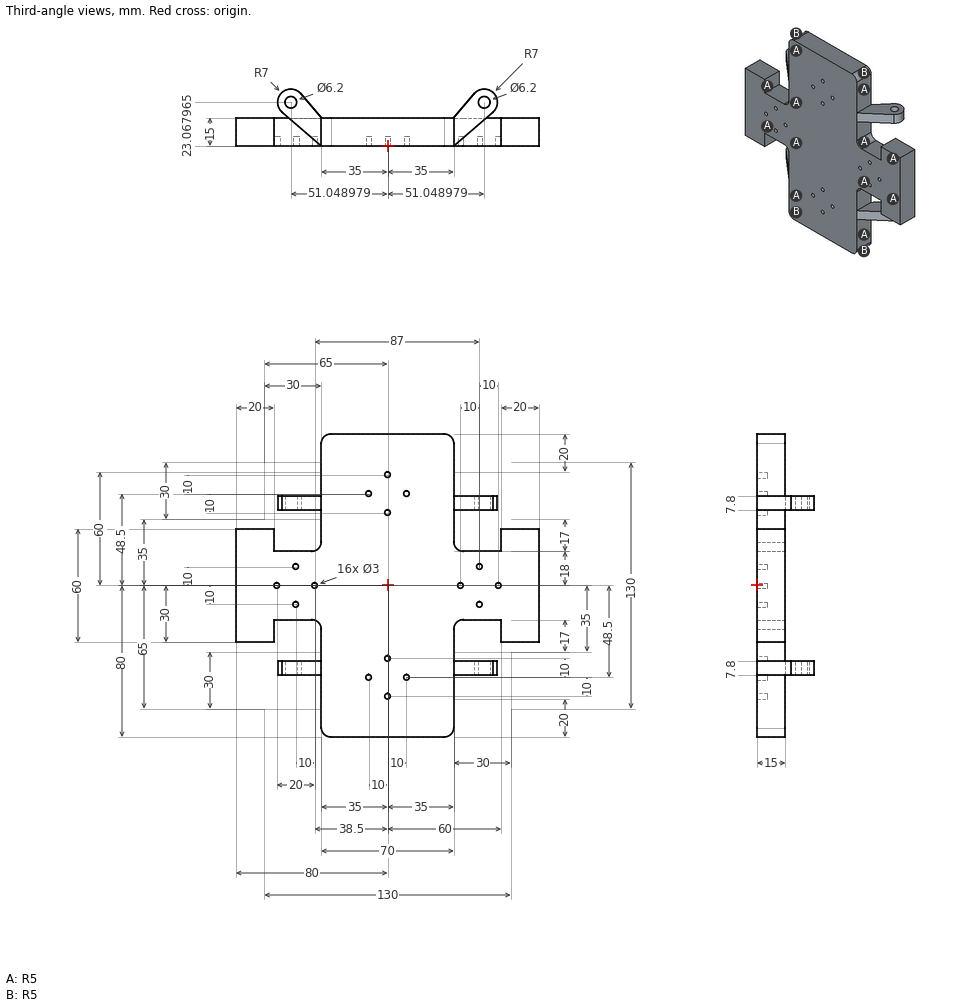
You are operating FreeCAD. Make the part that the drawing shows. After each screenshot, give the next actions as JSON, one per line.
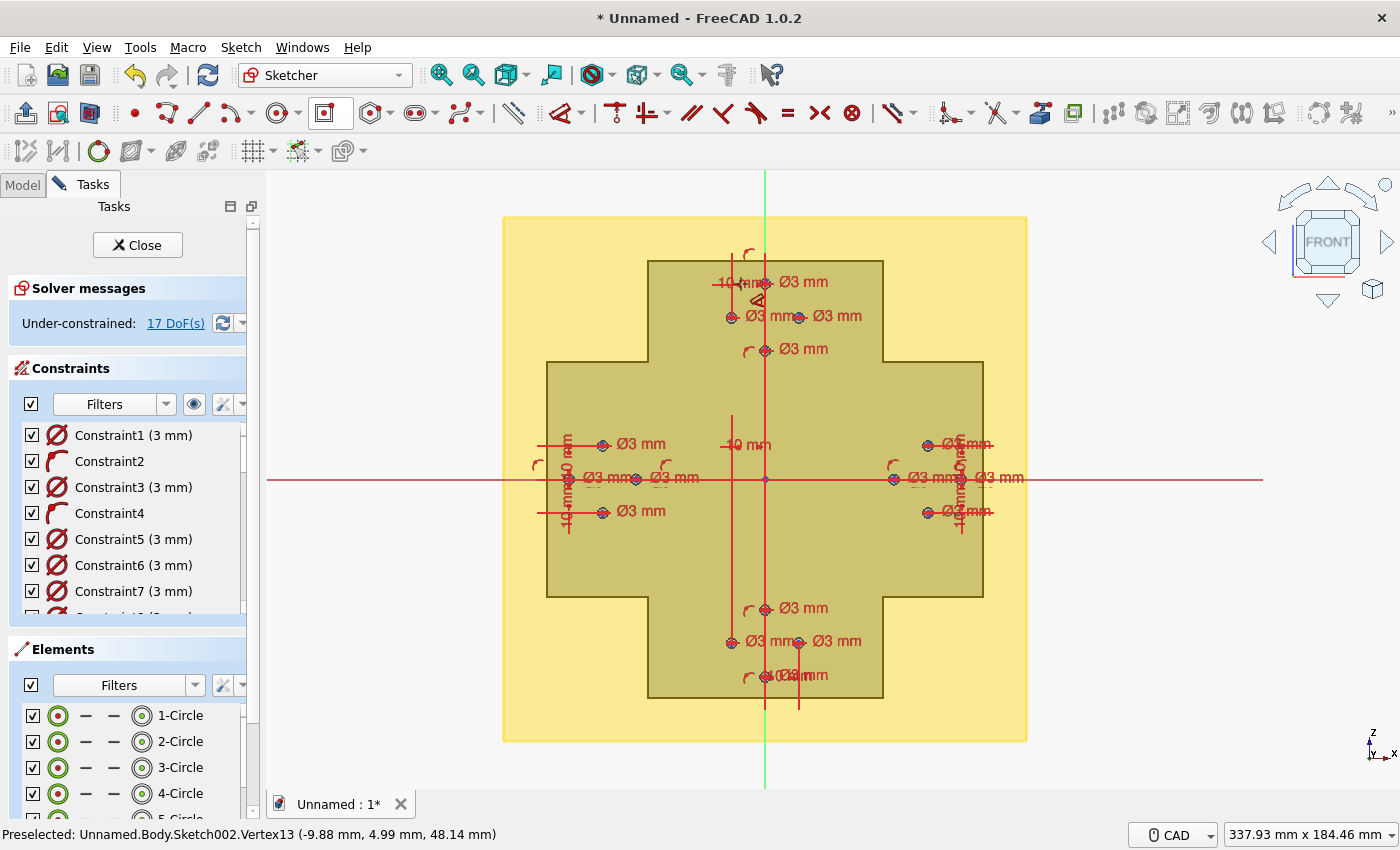
{"action": "left_click", "coordinate": [799, 318]}
{"action": "left_click", "coordinate": [782, 514]}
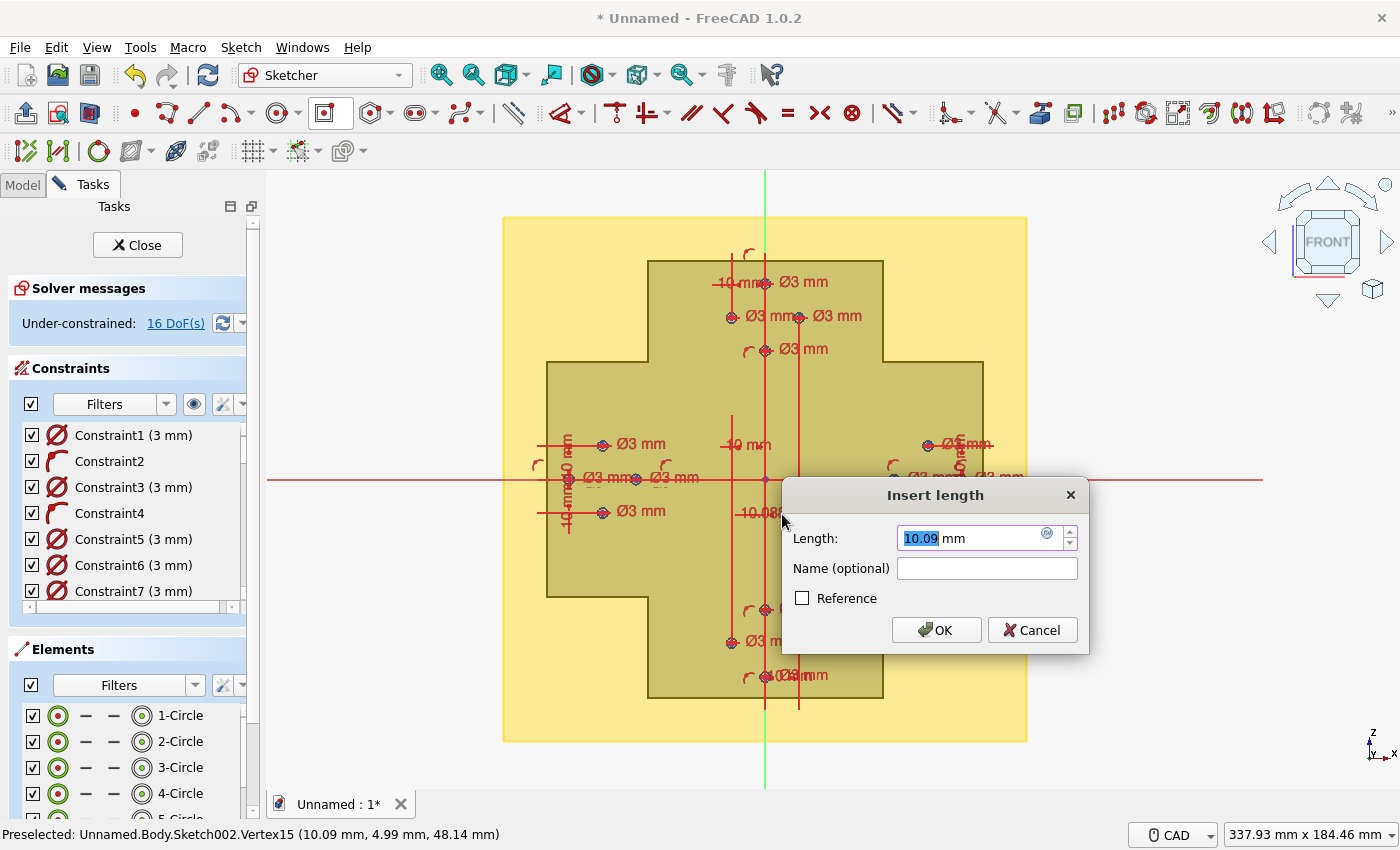
{"action": "type", "text": "10"}
{"action": "key", "text": "Return"}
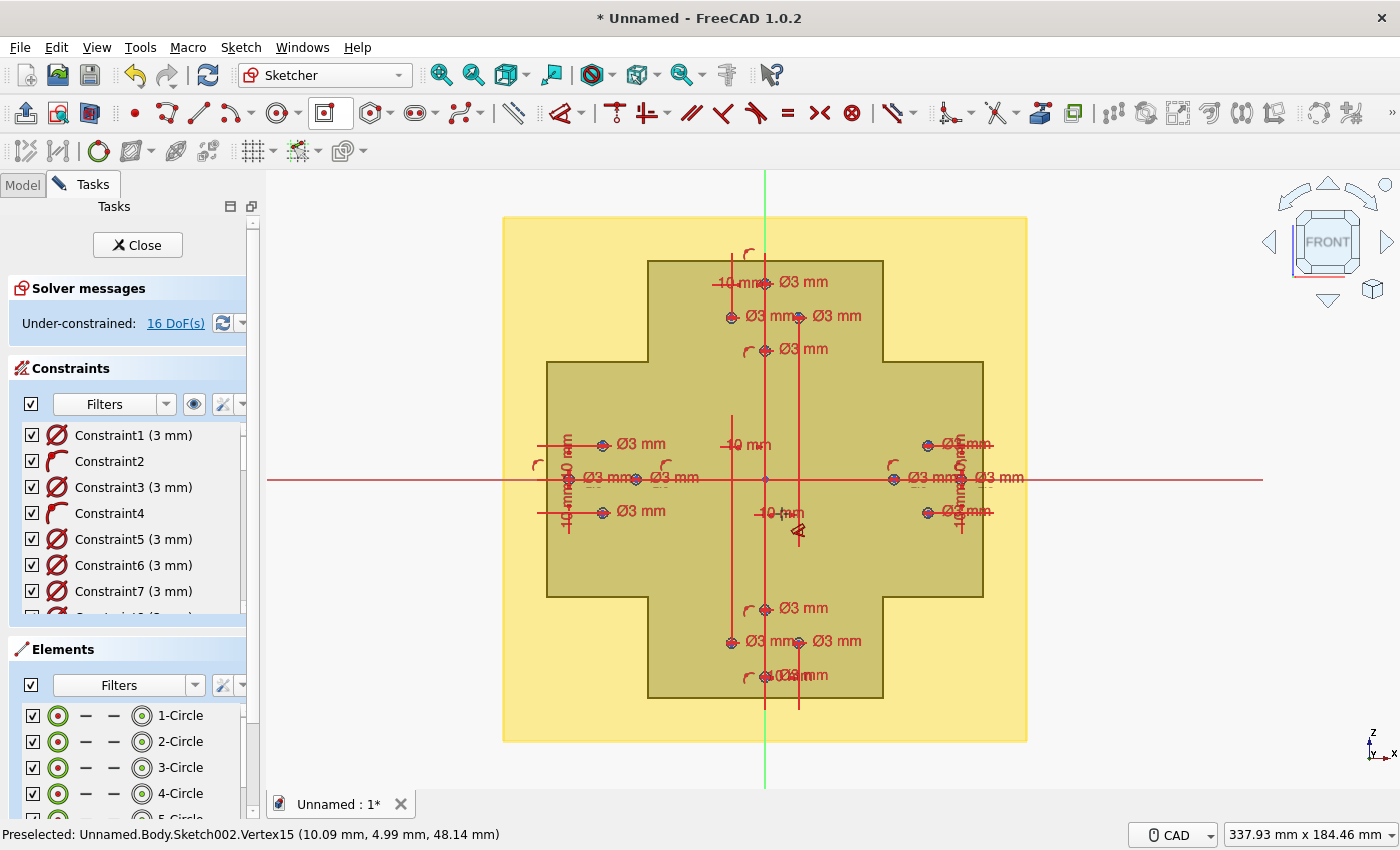
{"action": "left_click", "coordinate": [636, 480]}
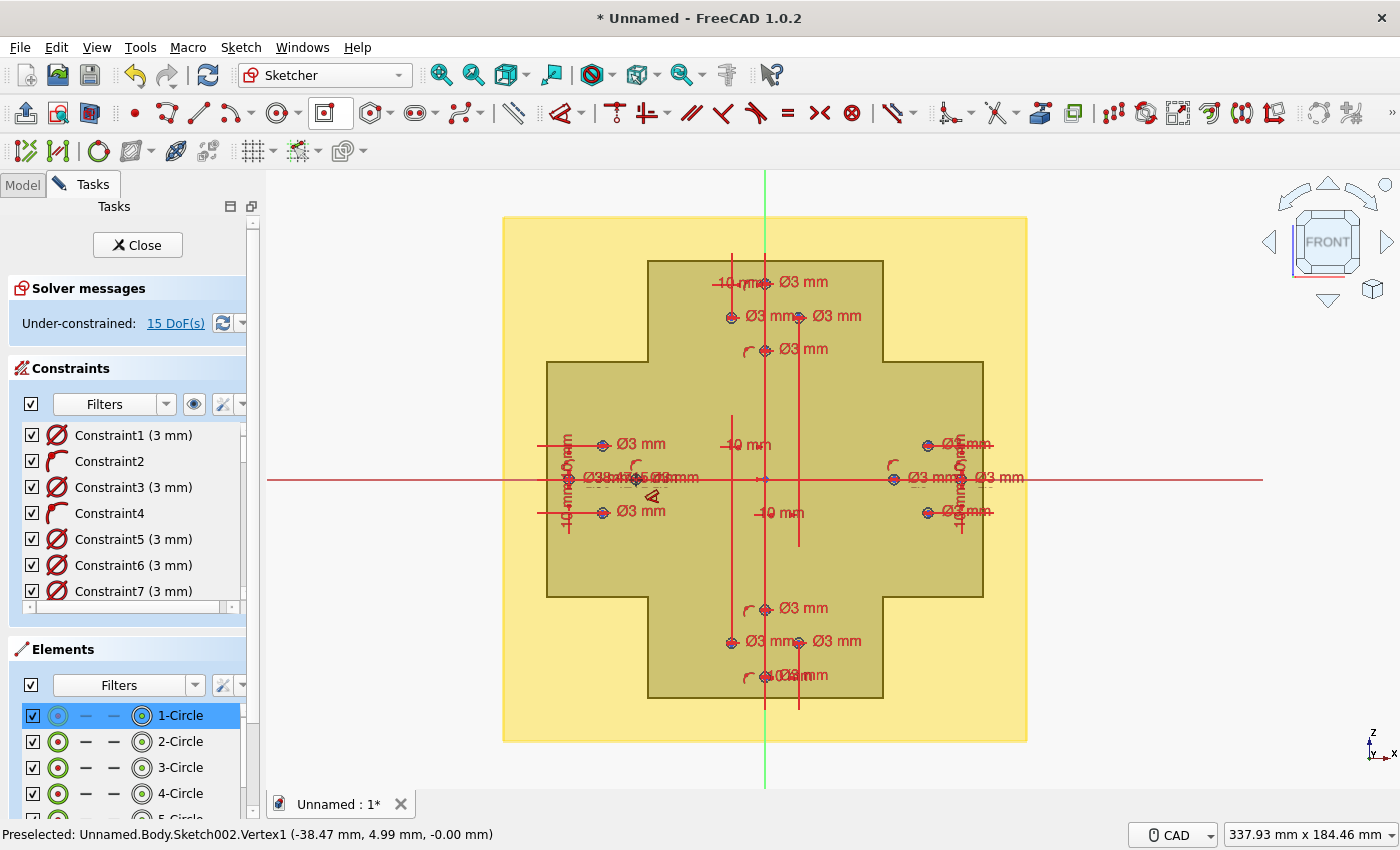
{"action": "left_click", "coordinate": [569, 480]}
{"action": "left_click", "coordinate": [603, 538]}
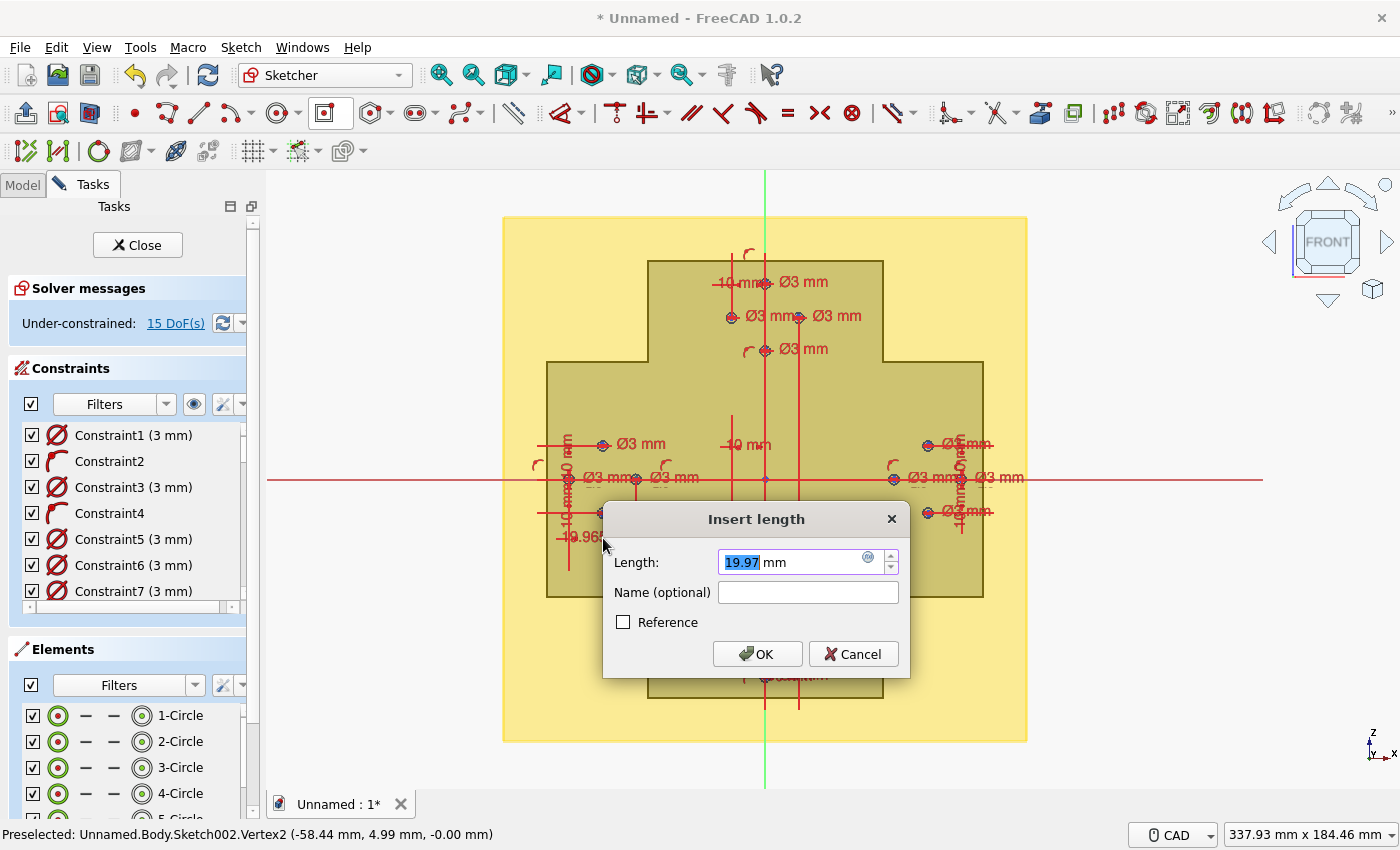
{"action": "type", "text": "20"}
{"action": "key", "text": "Return"}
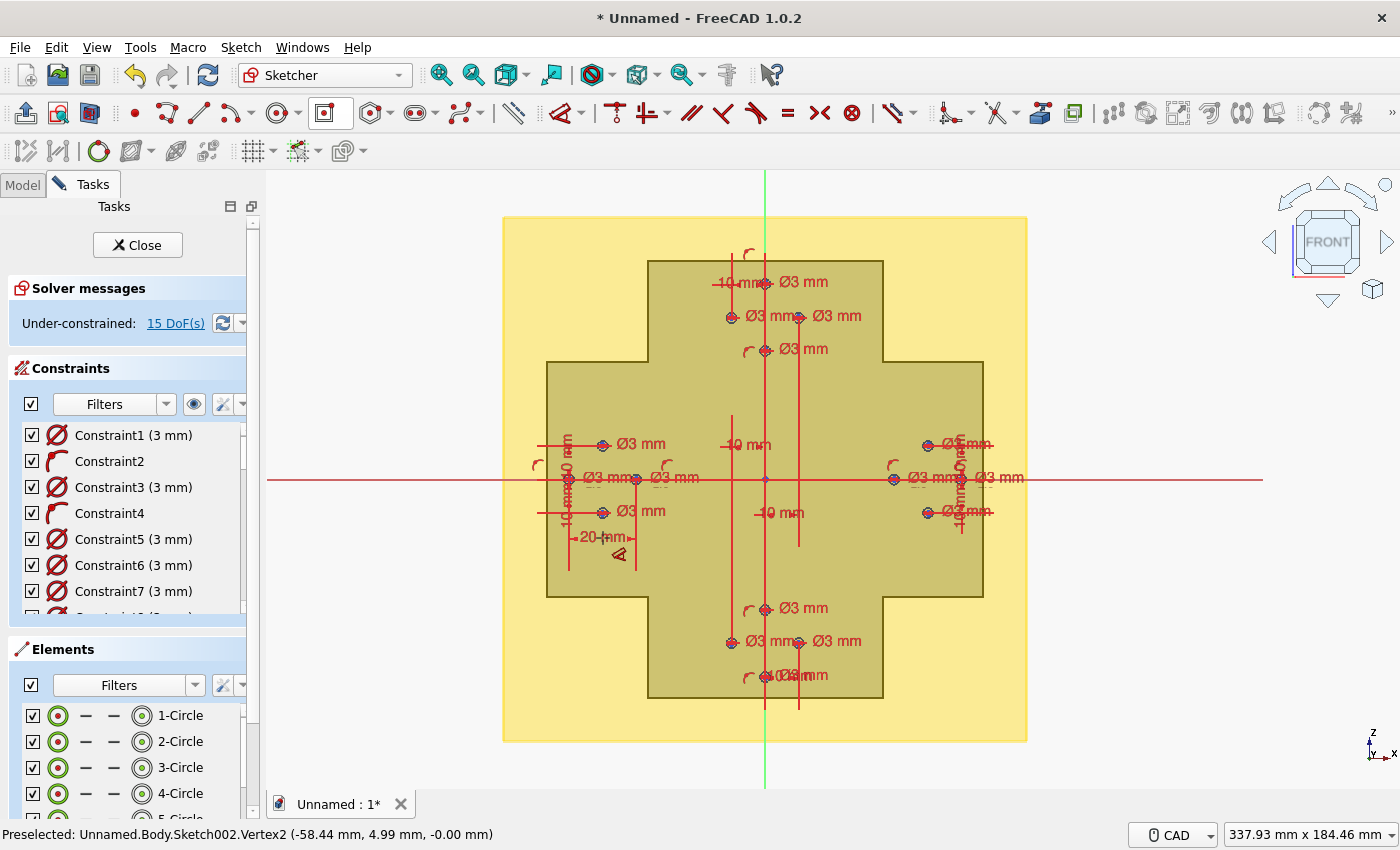
{"action": "left_click", "coordinate": [636, 480]}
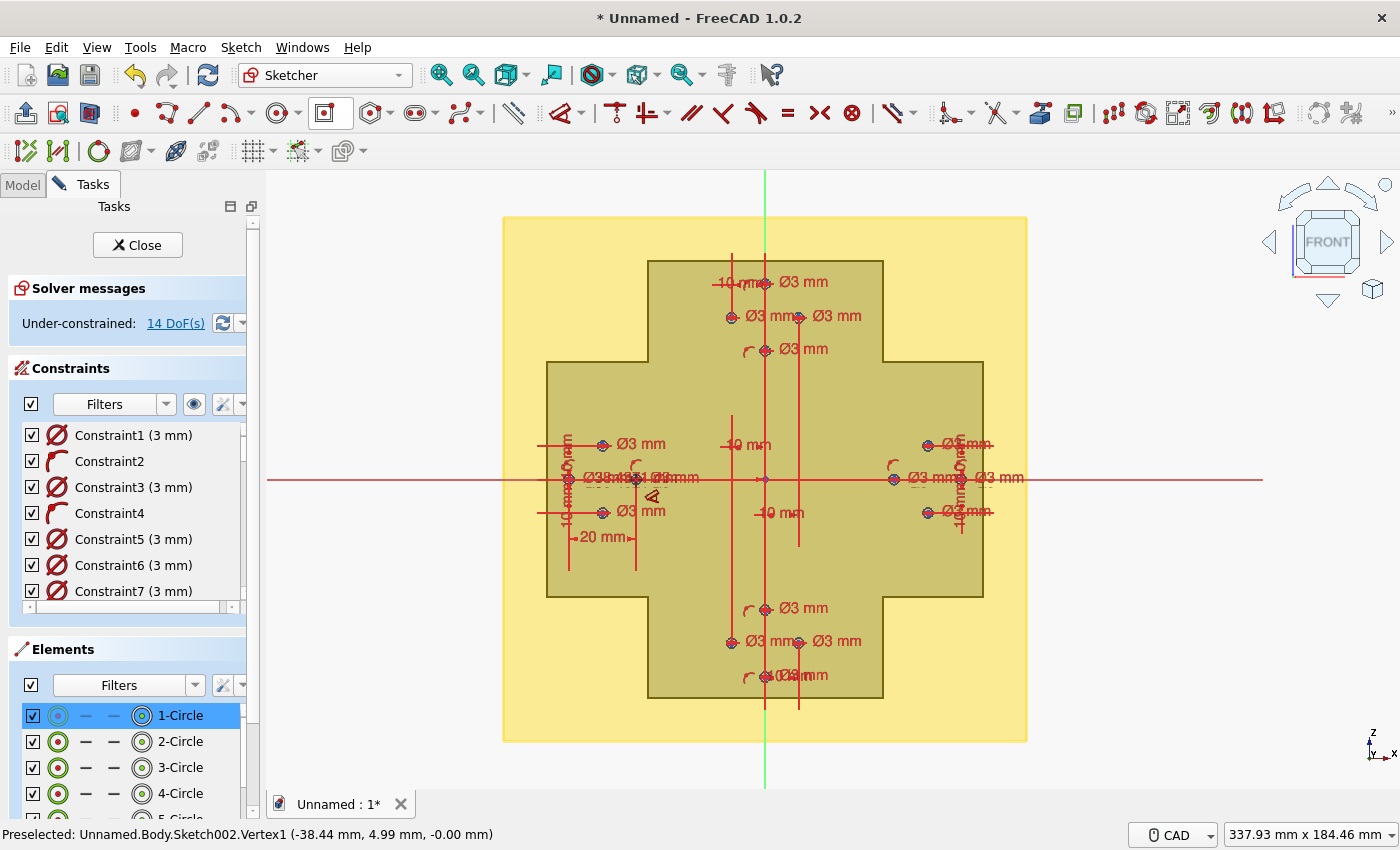
{"action": "left_click", "coordinate": [603, 513]}
{"action": "left_click", "coordinate": [619, 571]}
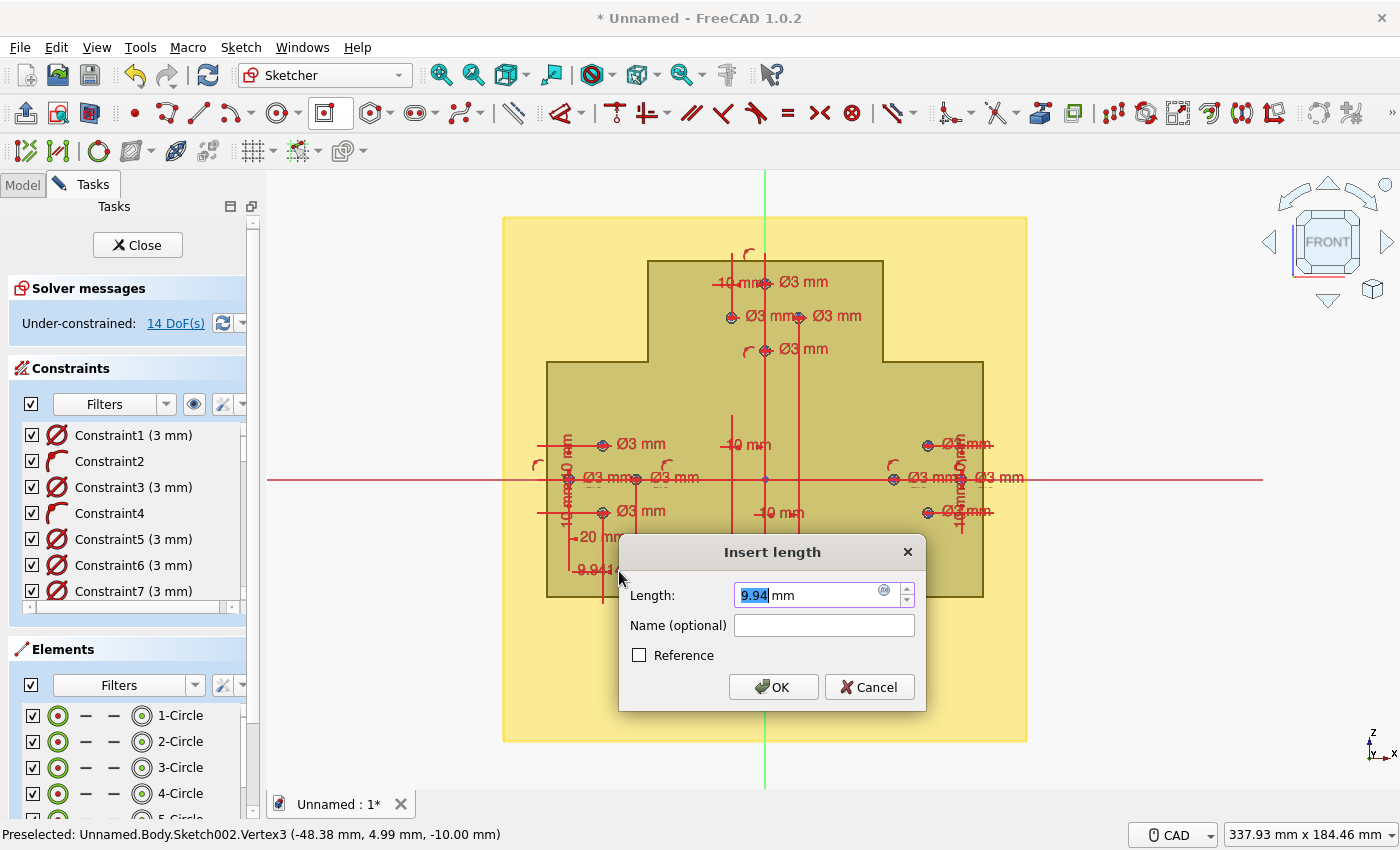
{"action": "type", "text": "10"}
{"action": "key", "text": "Return"}